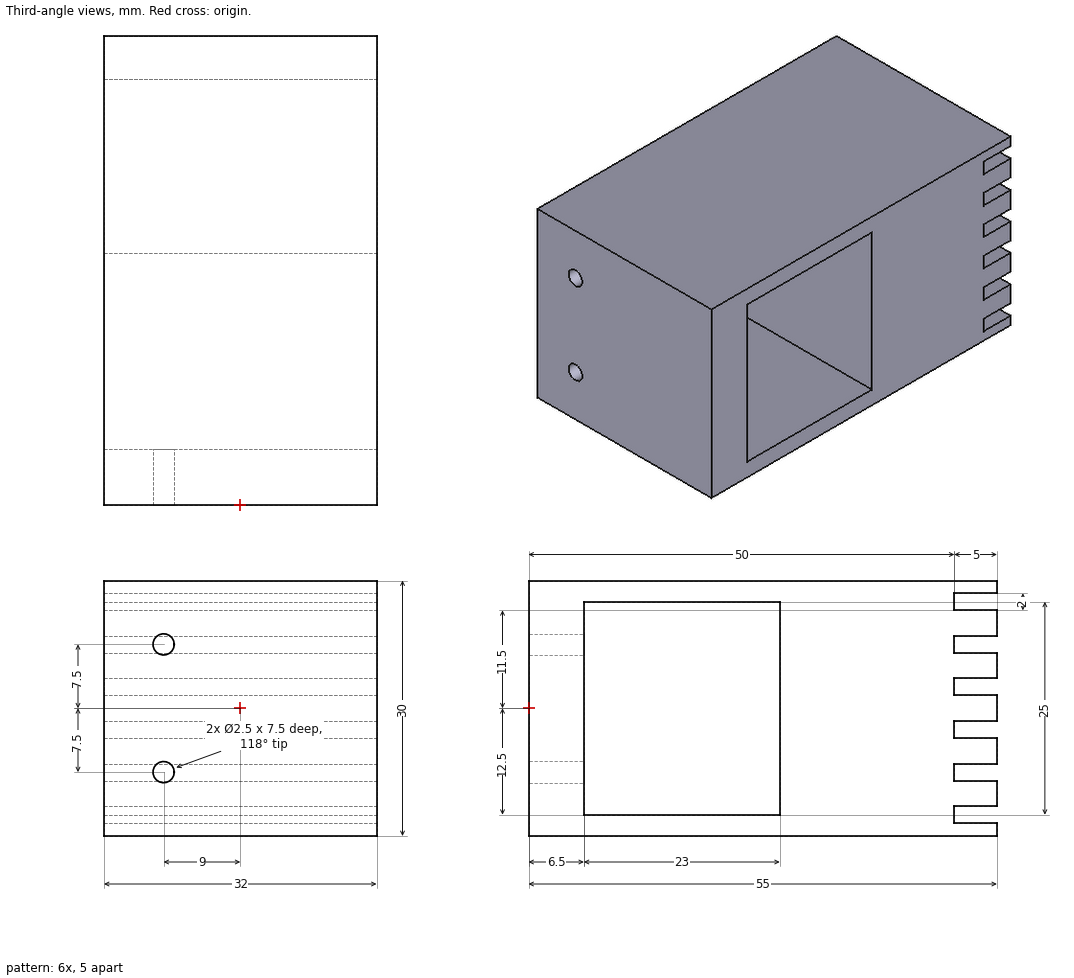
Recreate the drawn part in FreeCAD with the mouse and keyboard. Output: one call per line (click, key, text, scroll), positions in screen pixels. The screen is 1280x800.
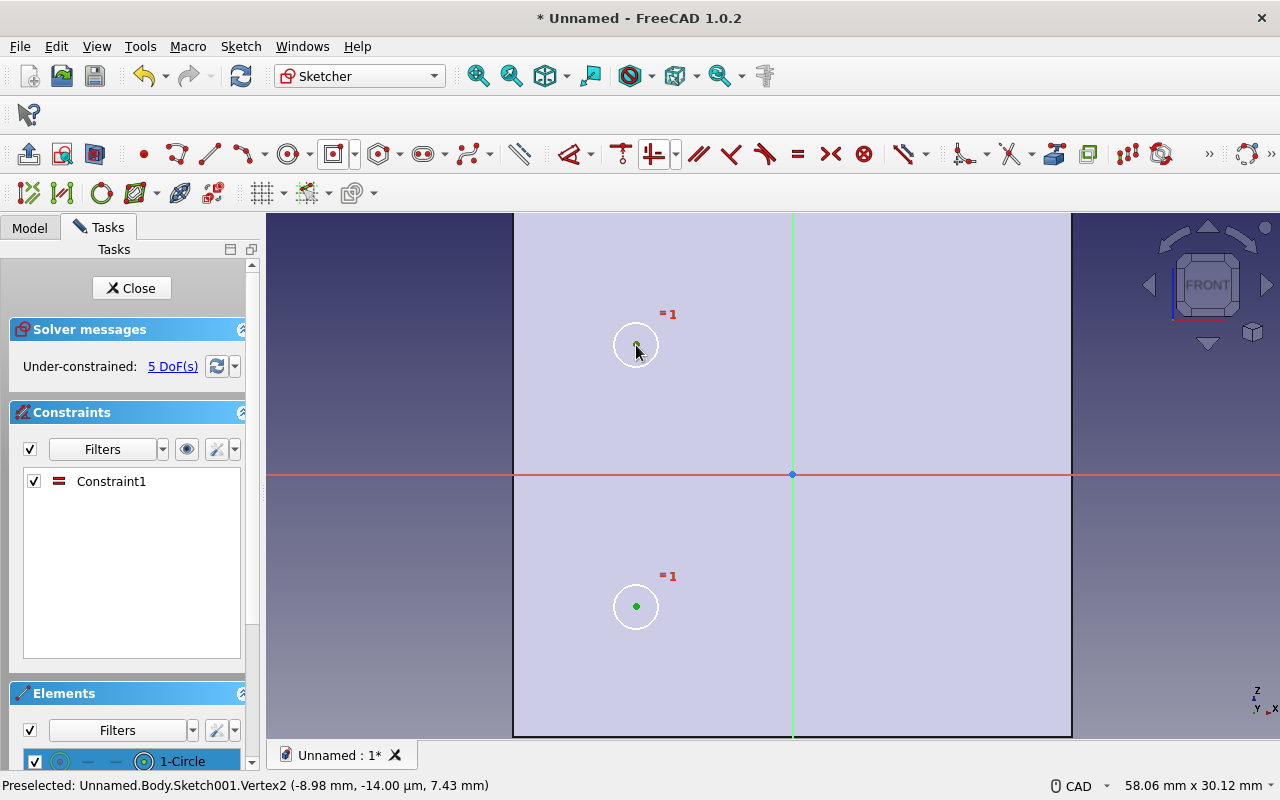
key(v)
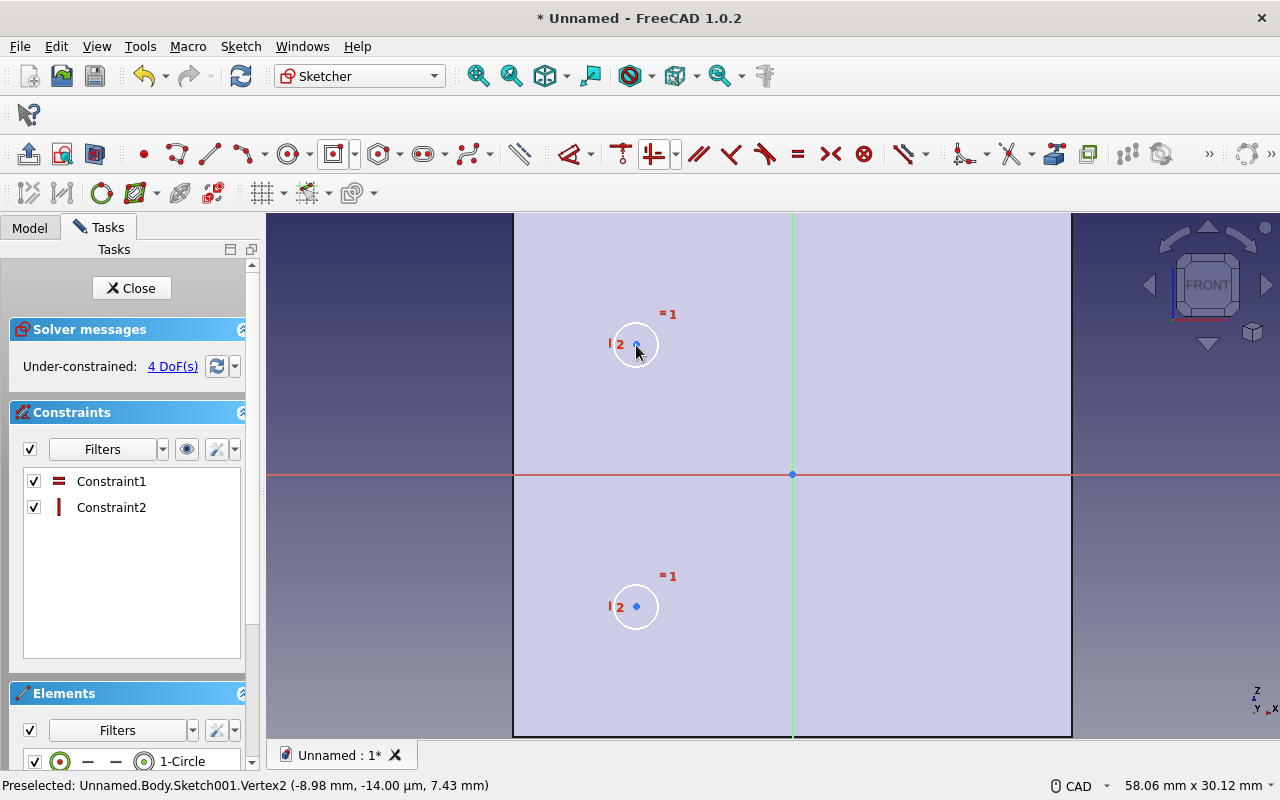
click(568, 154)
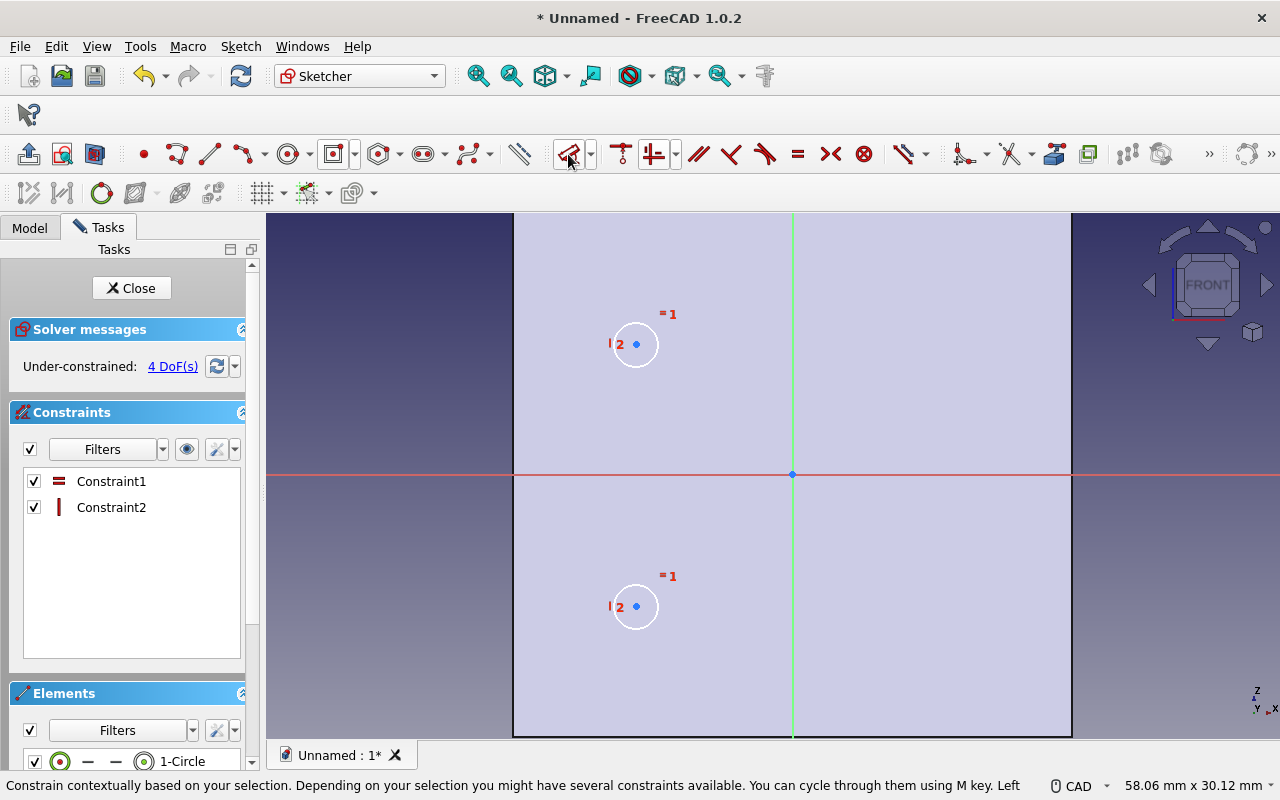
click(651, 591)
click(673, 568)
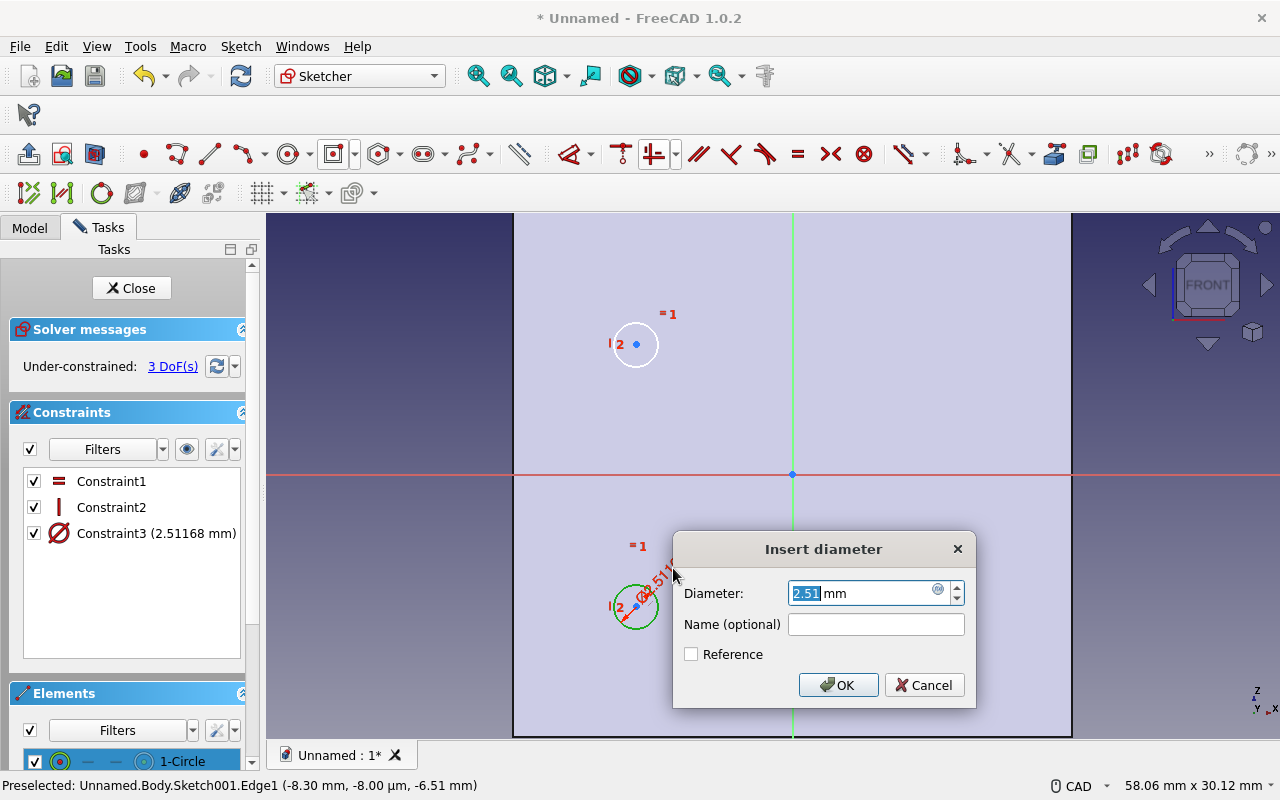
text(2.5)
key(Return)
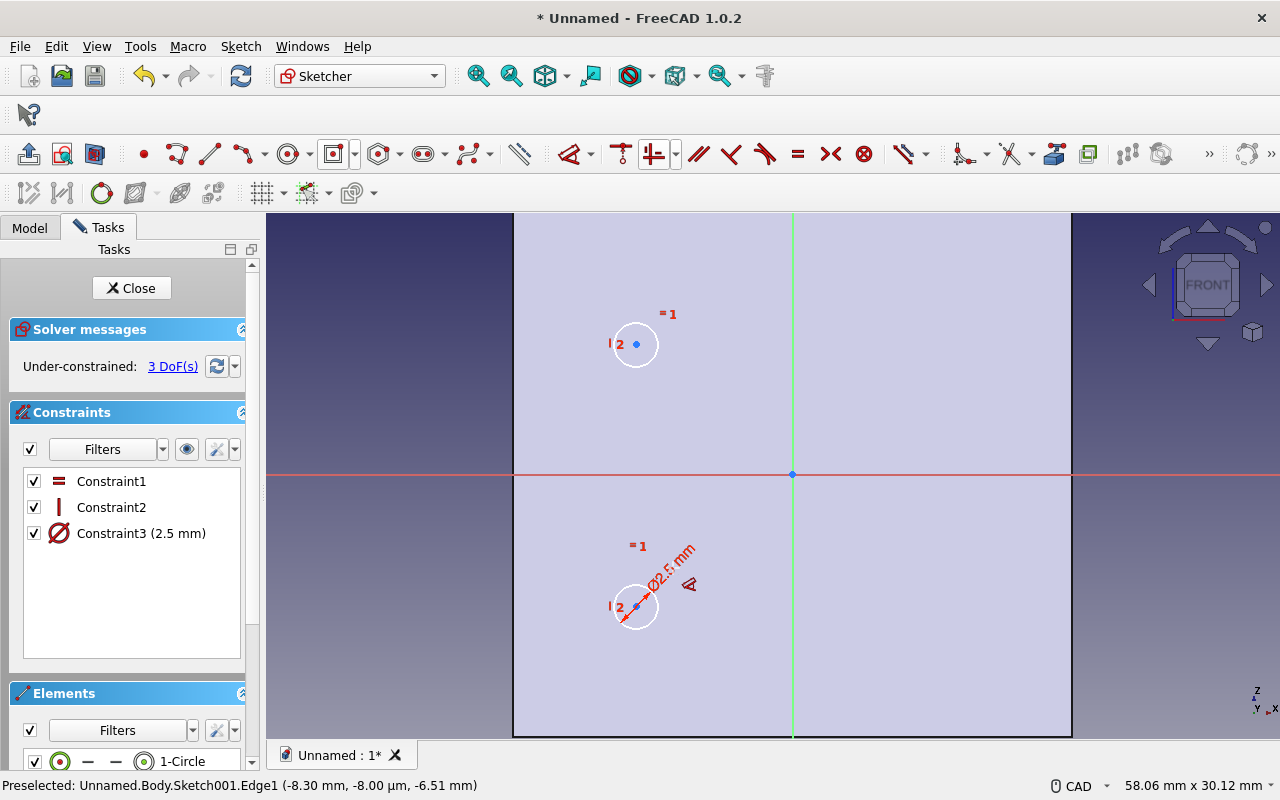
click(636, 607)
click(714, 641)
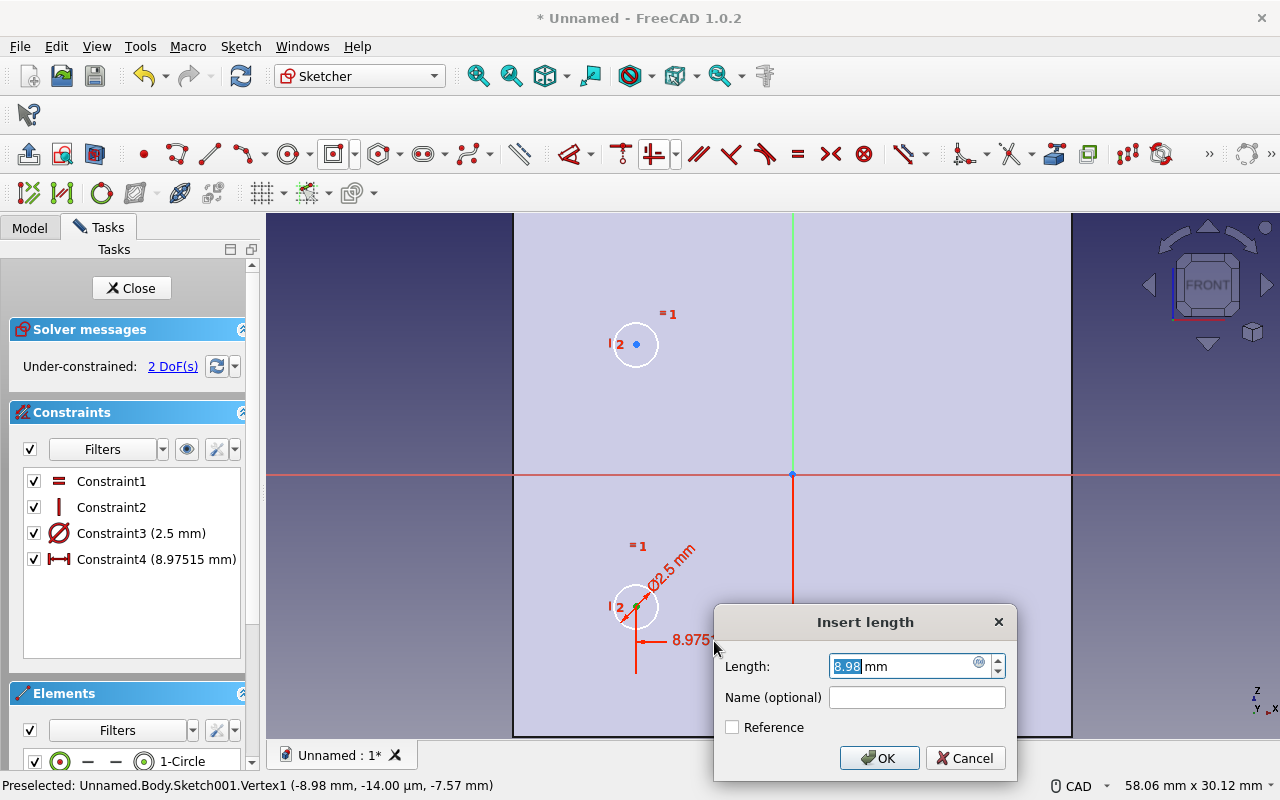
text(9)
key(Return)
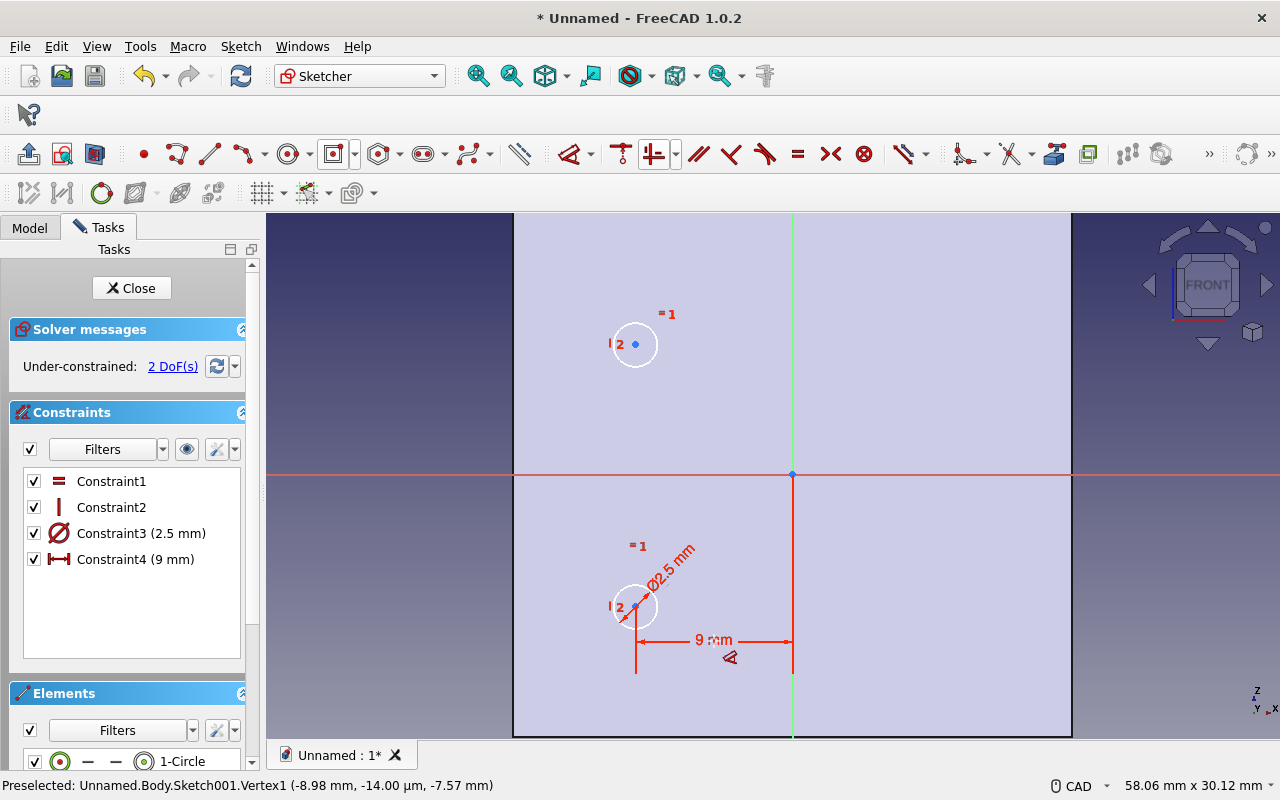
click(636, 607)
click(827, 541)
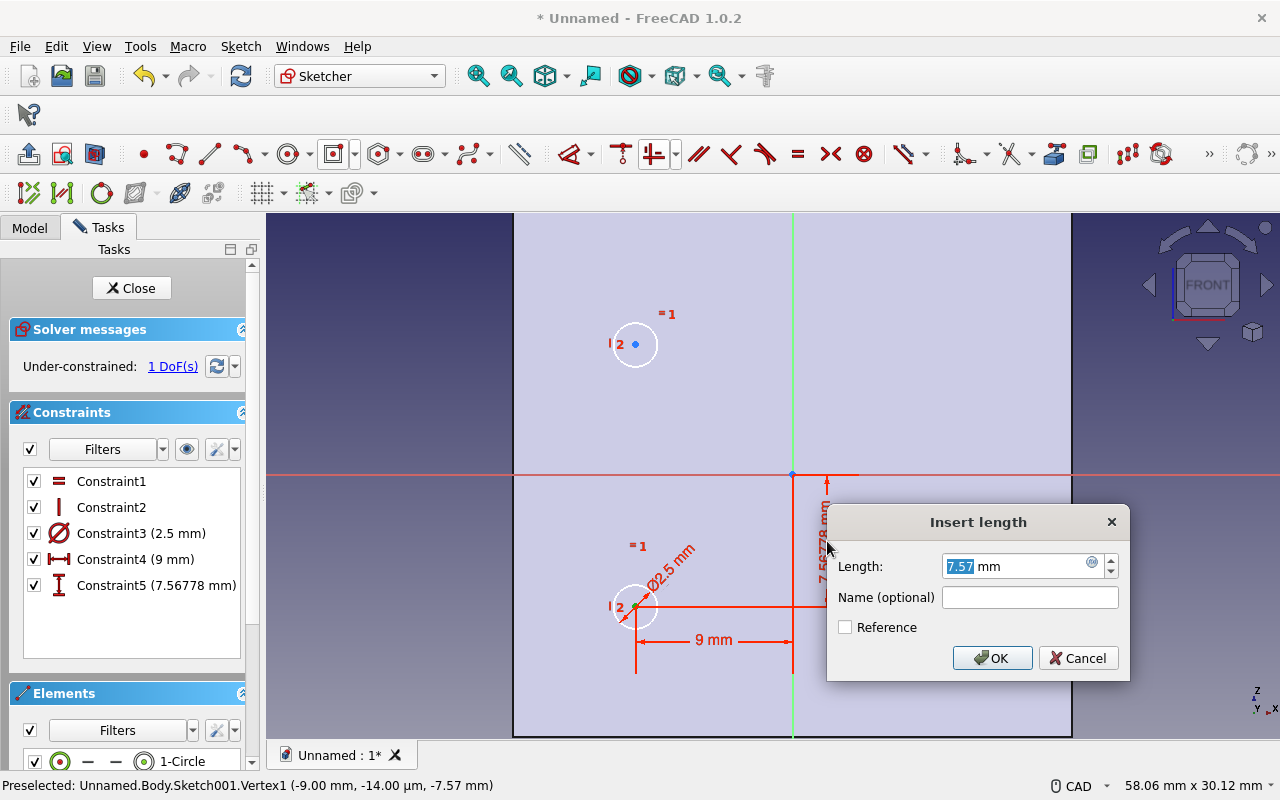
text(7.5)
key(Return)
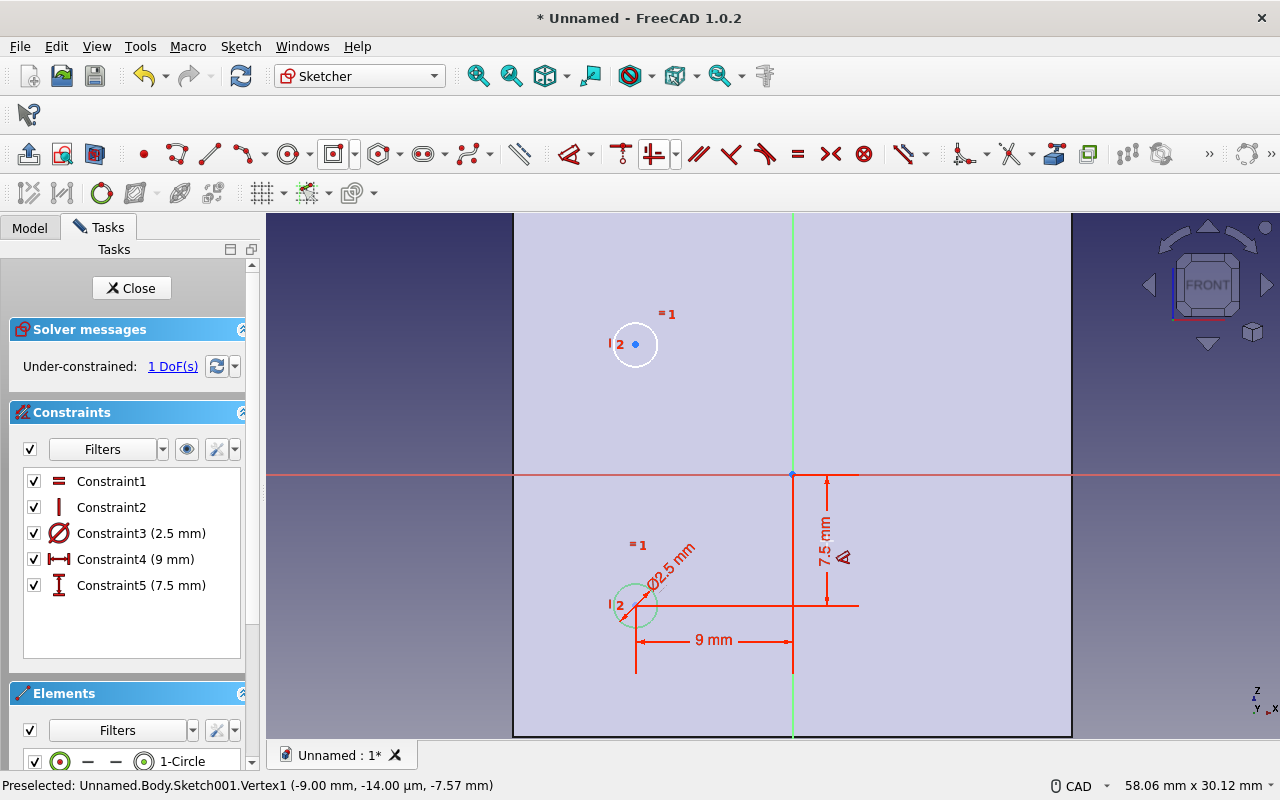
click(636, 345)
click(827, 410)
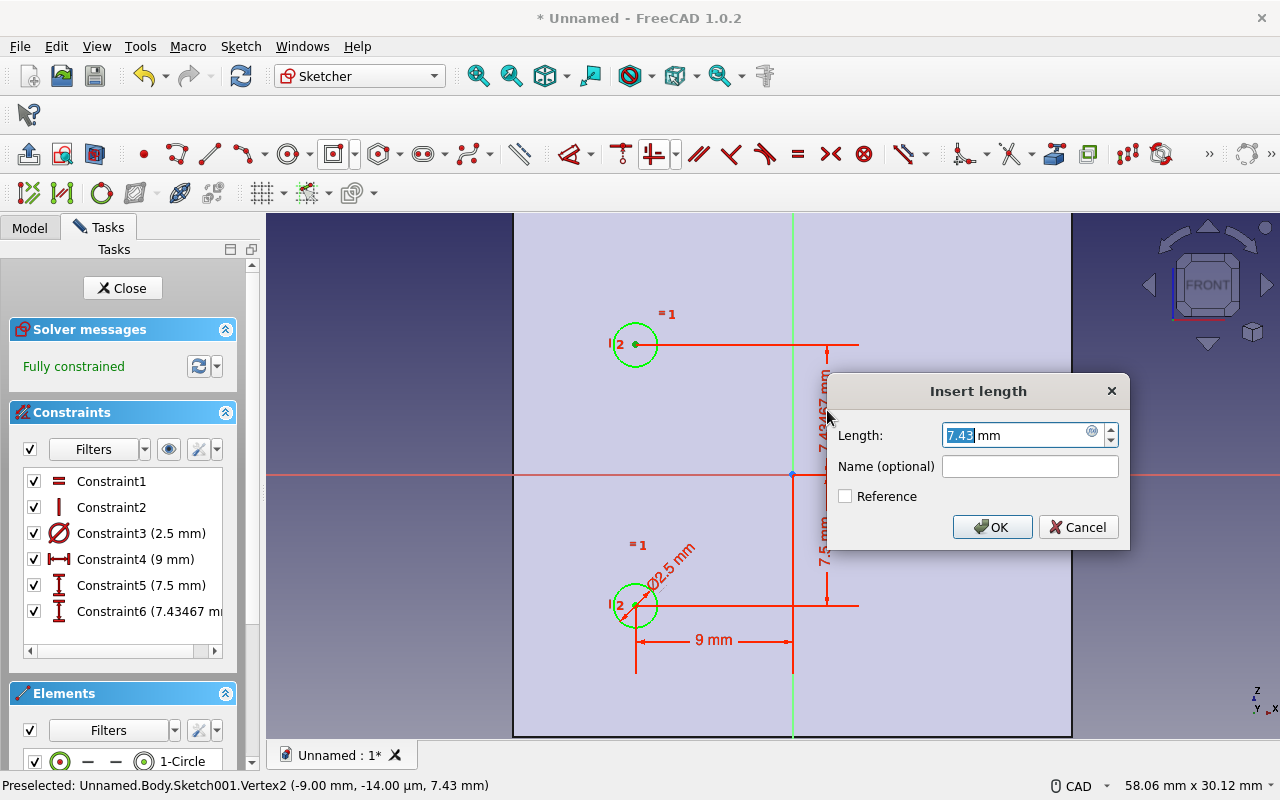
text(7.5)
key(Return)
key(Escape)